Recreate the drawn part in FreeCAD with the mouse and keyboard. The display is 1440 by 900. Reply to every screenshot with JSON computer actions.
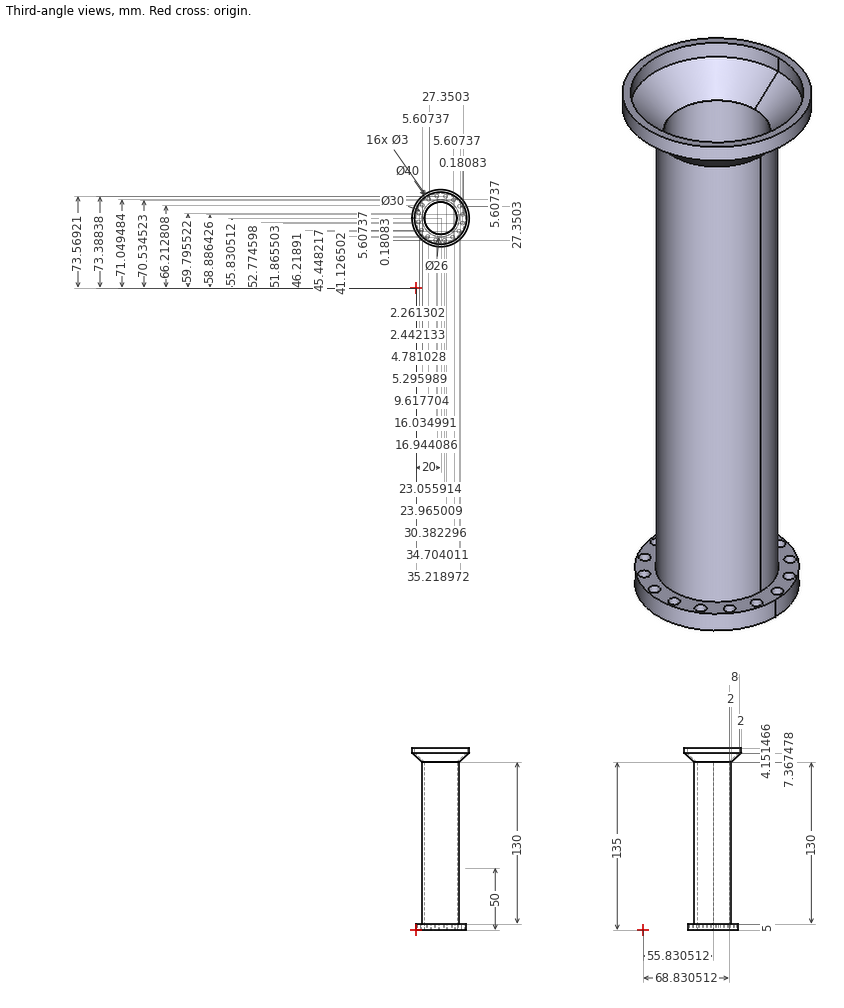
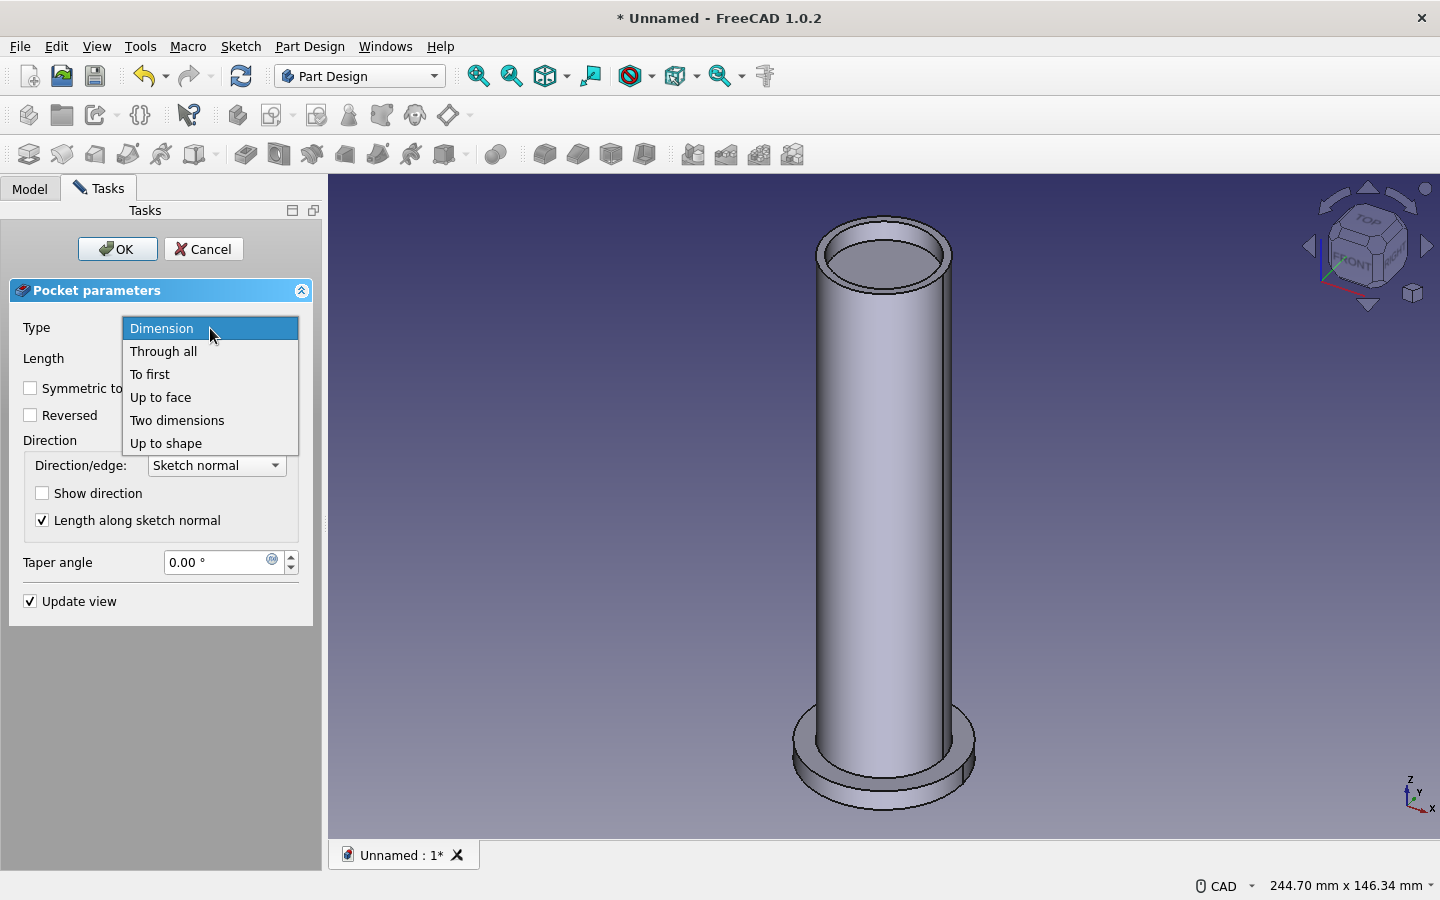
{"action": "left_click", "coordinate": [208, 420]}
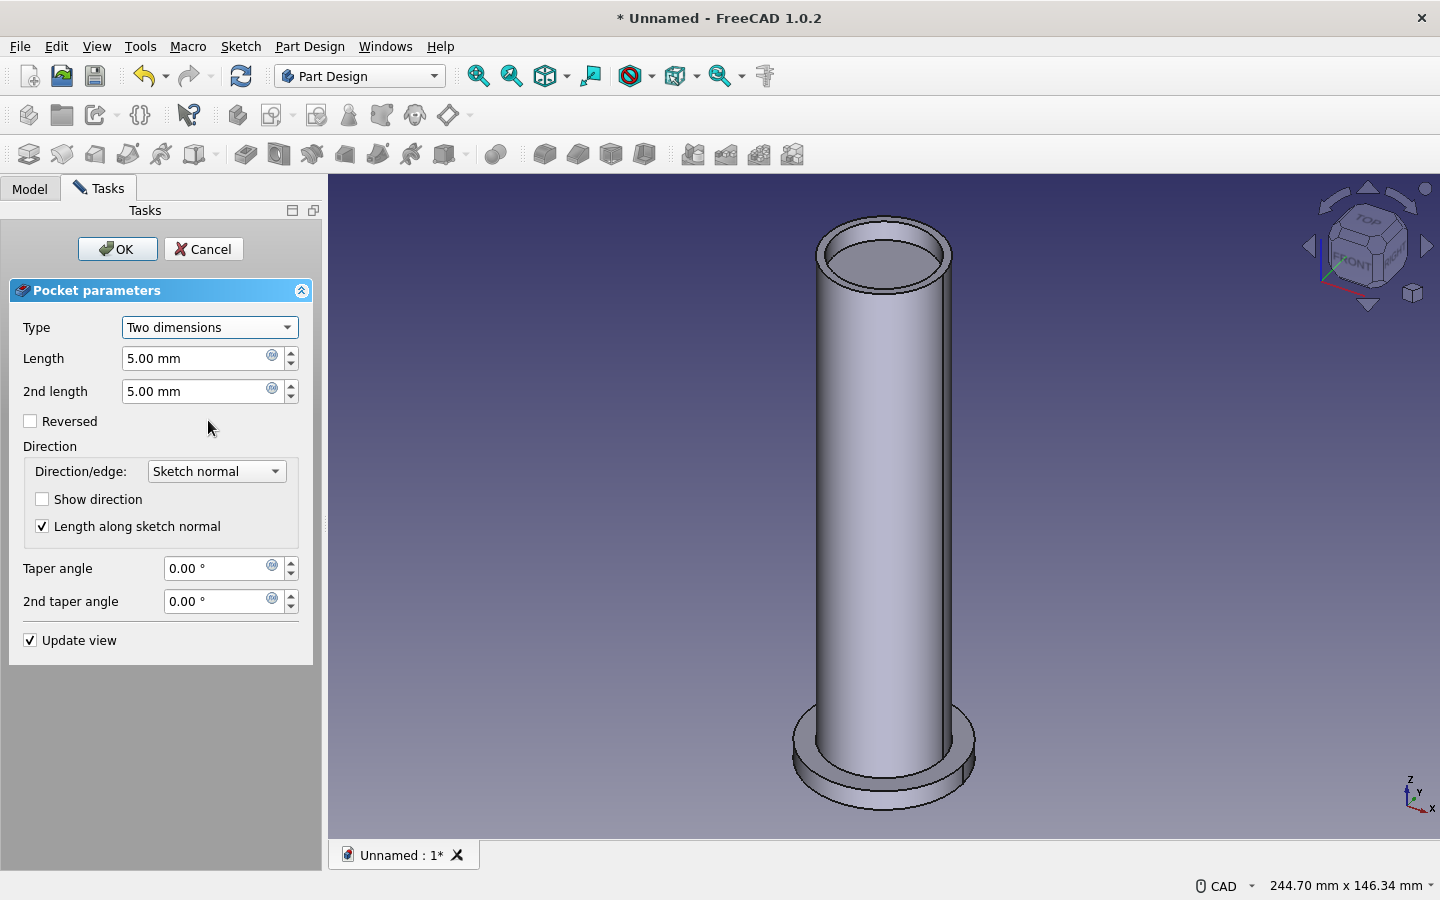
{"action": "triple_click", "coordinate": [204, 358]}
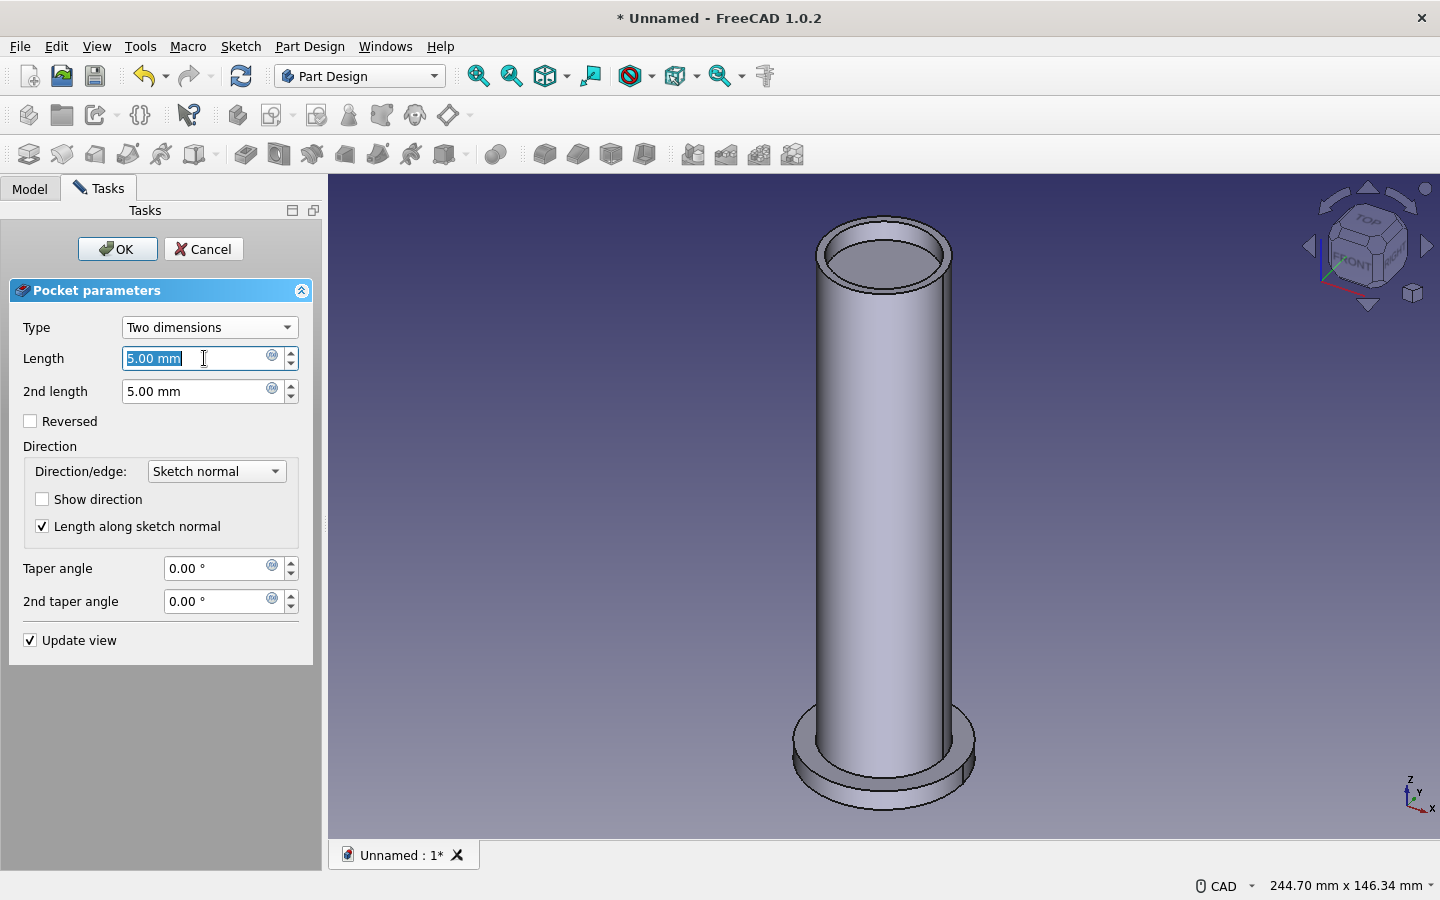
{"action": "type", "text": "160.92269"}
{"action": "key", "text": "Tab"}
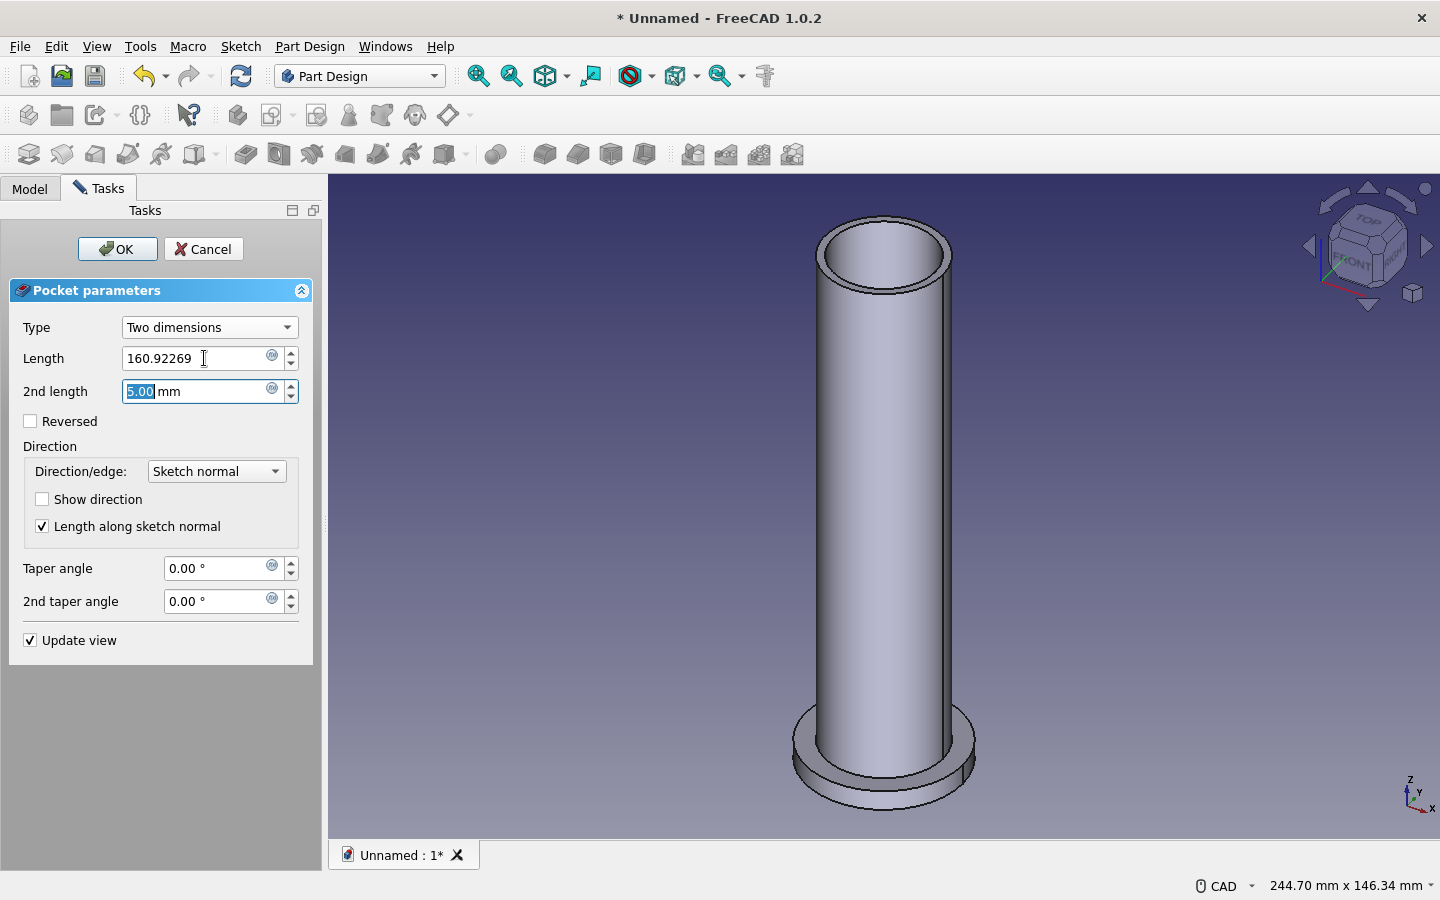
{"action": "type", "text": "130"}
{"action": "key", "text": "Tab"}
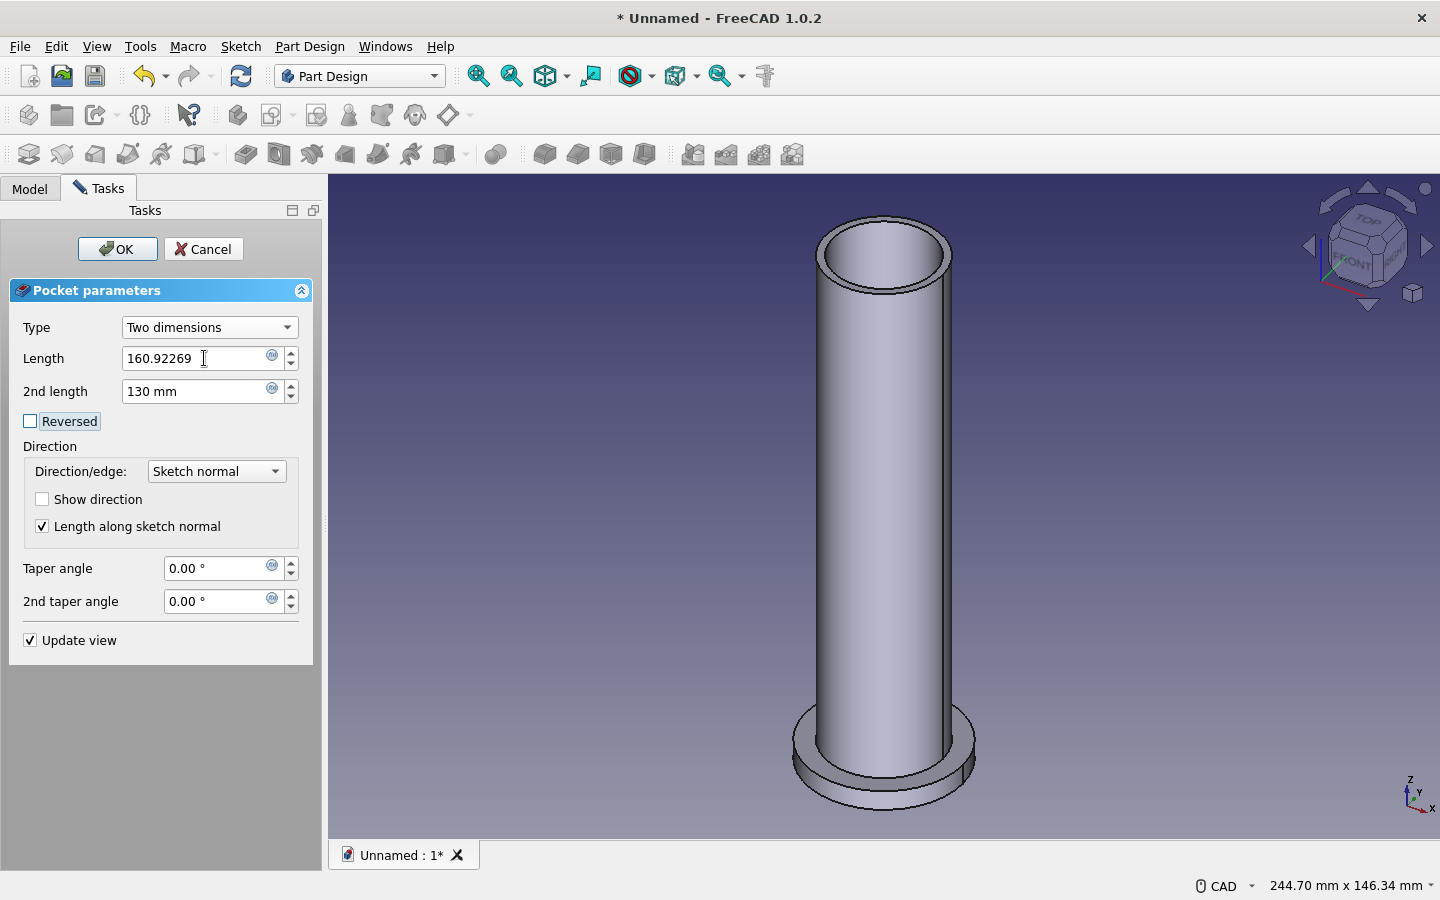
{"action": "left_click", "coordinate": [31, 421]}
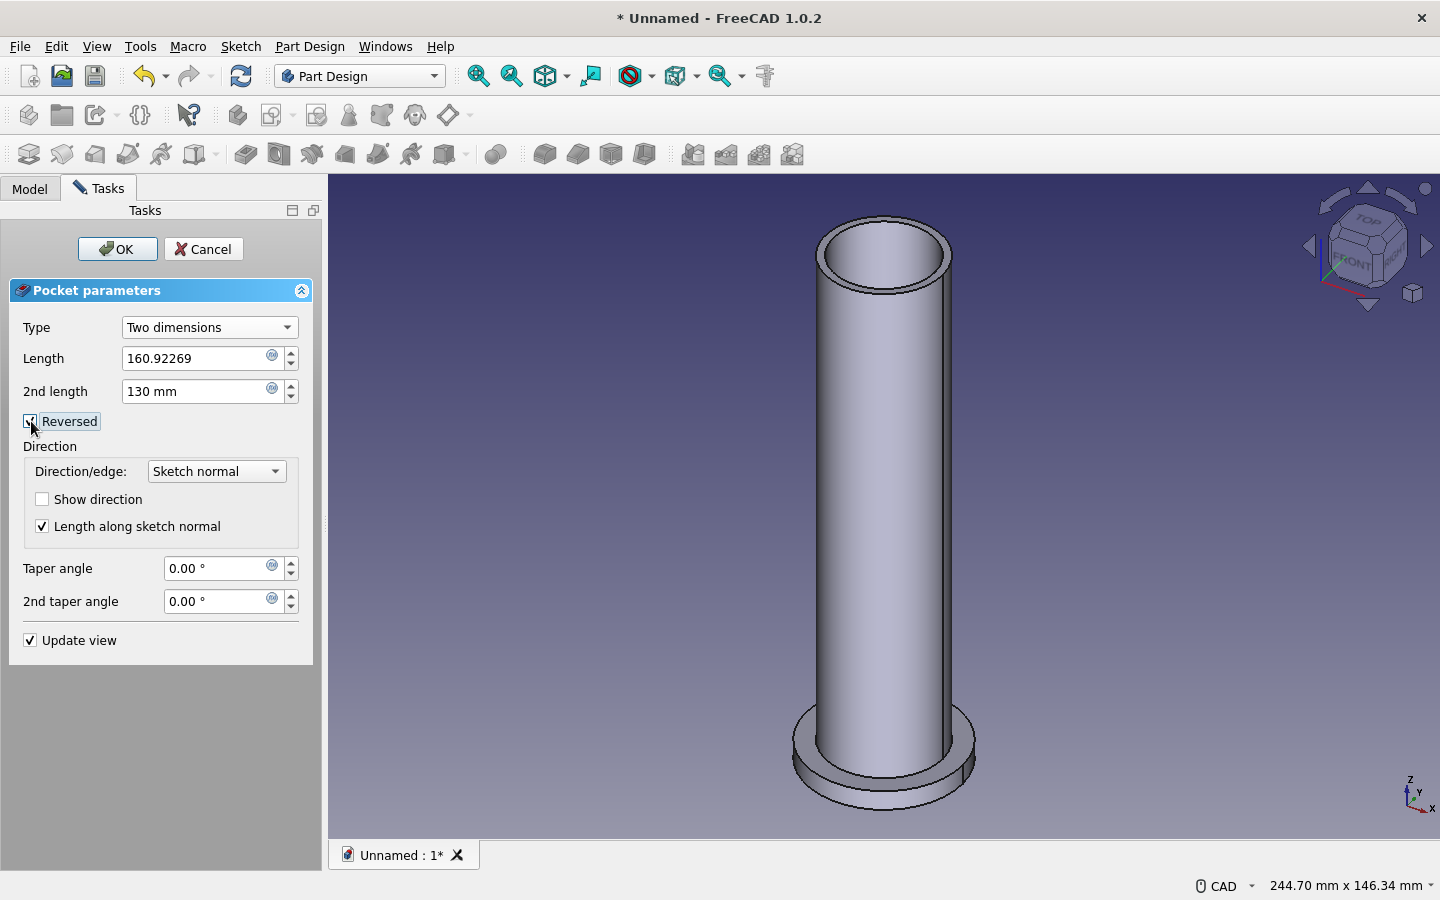
{"action": "left_click", "coordinate": [118, 249]}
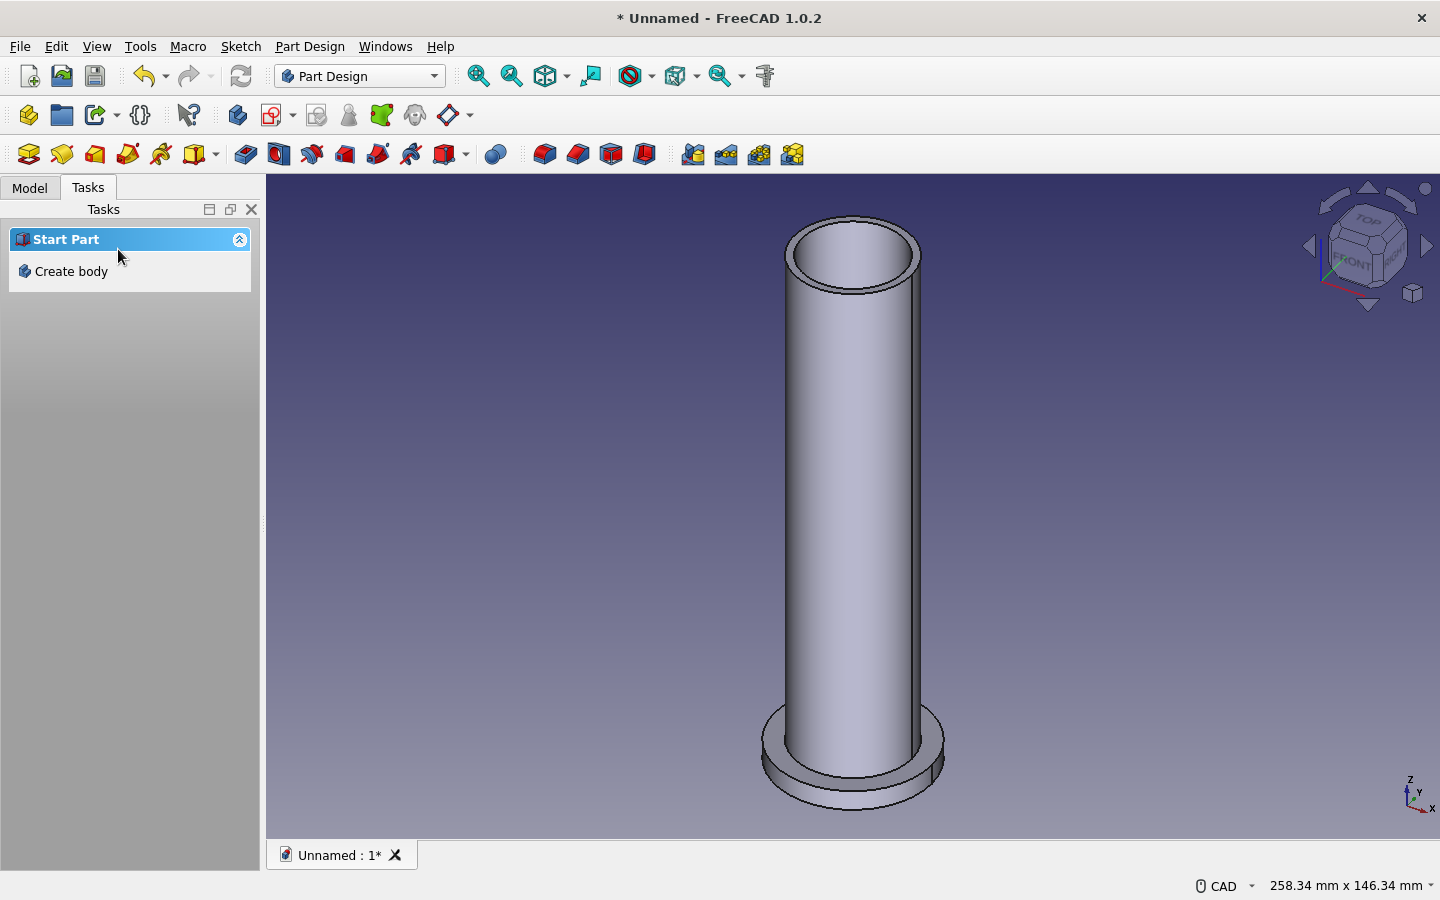
{"action": "key", "text": "0"}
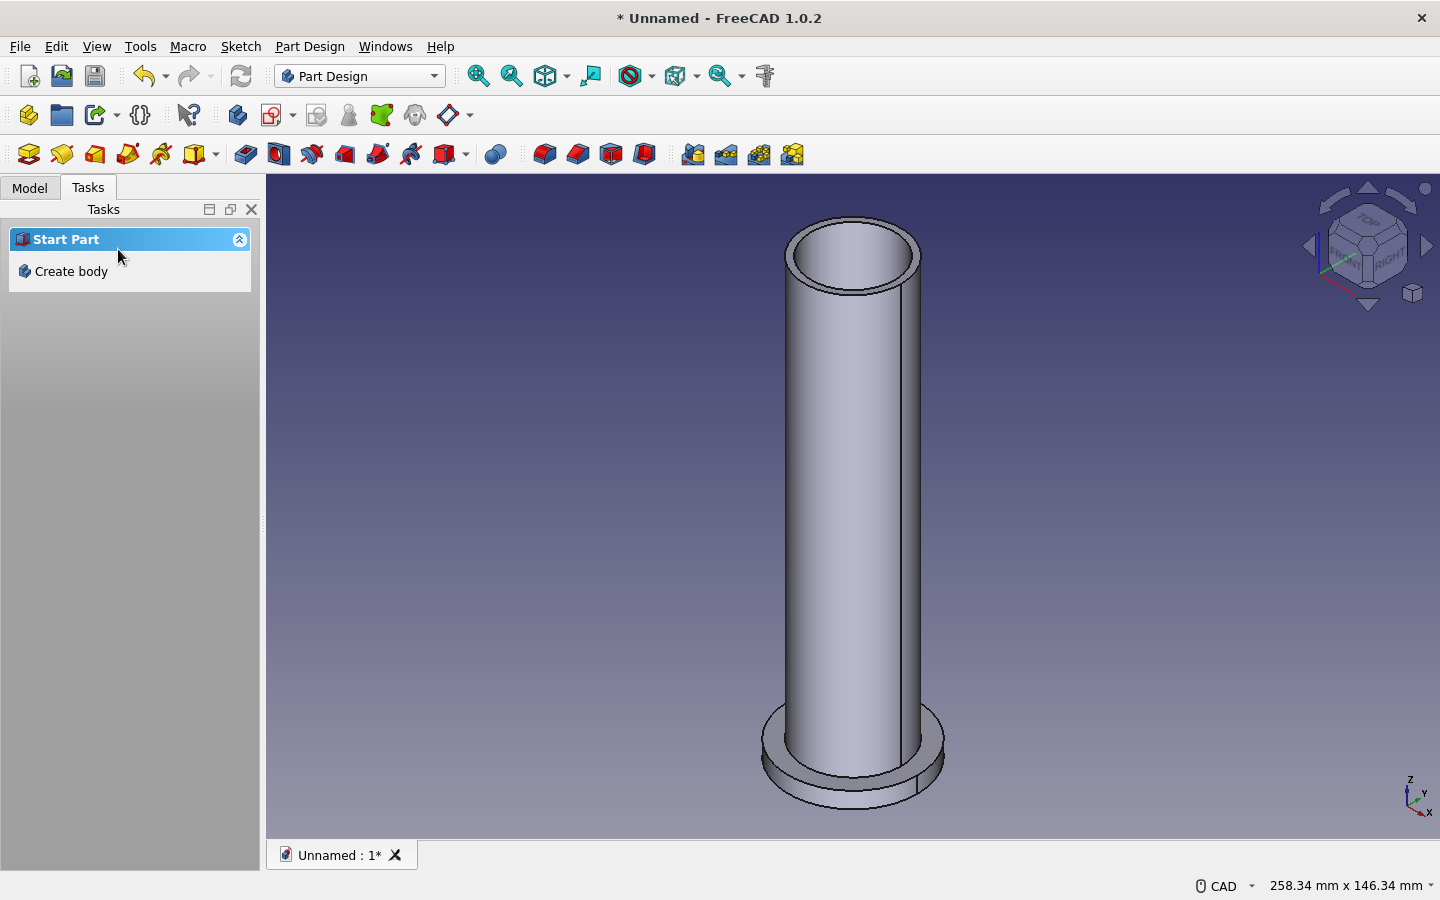
{"action": "left_click", "coordinate": [908, 769]}